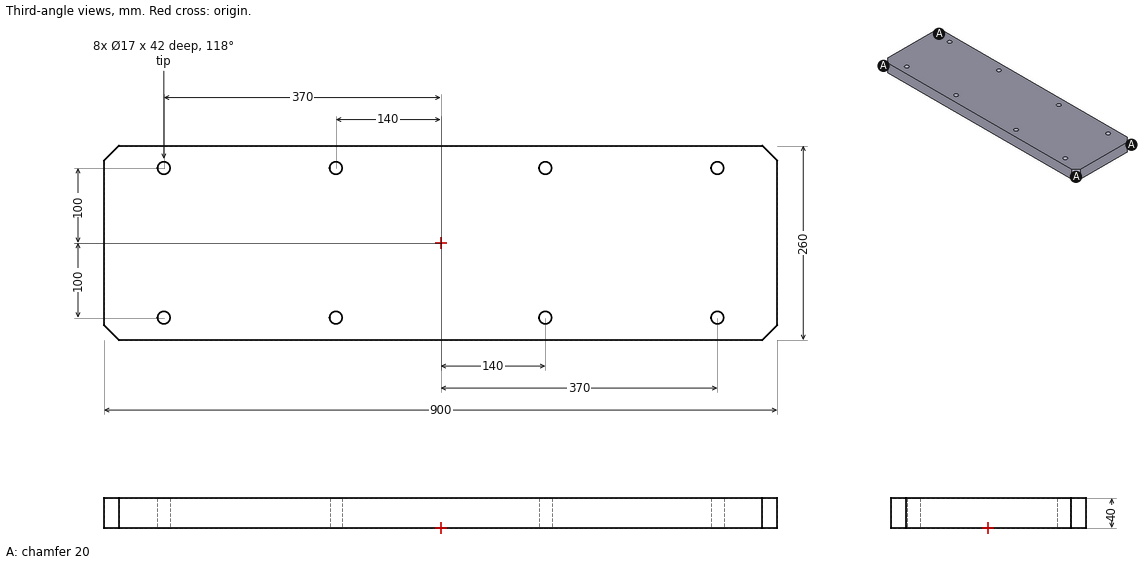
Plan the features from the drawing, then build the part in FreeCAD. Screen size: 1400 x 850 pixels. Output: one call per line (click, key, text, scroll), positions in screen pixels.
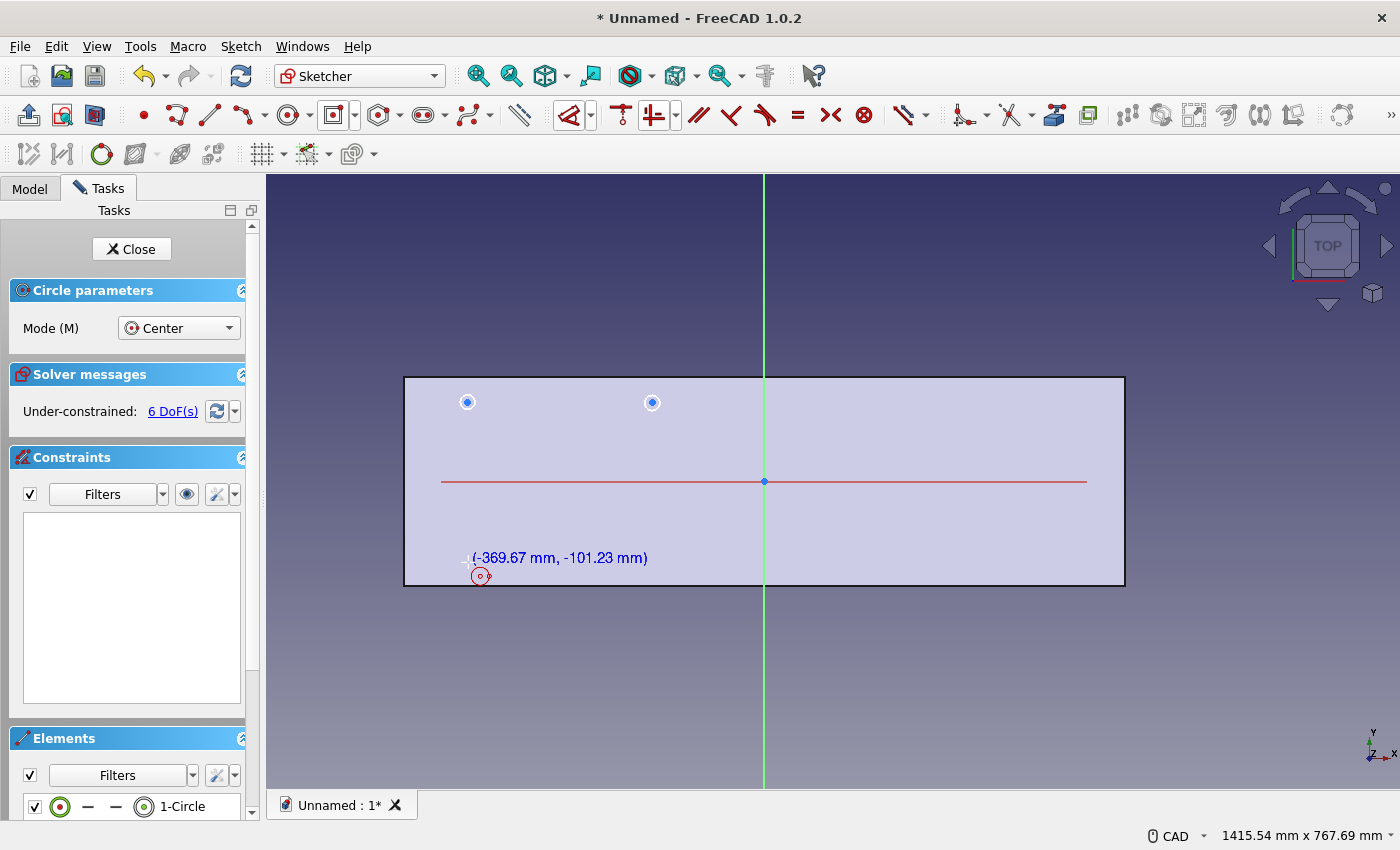
click(468, 562)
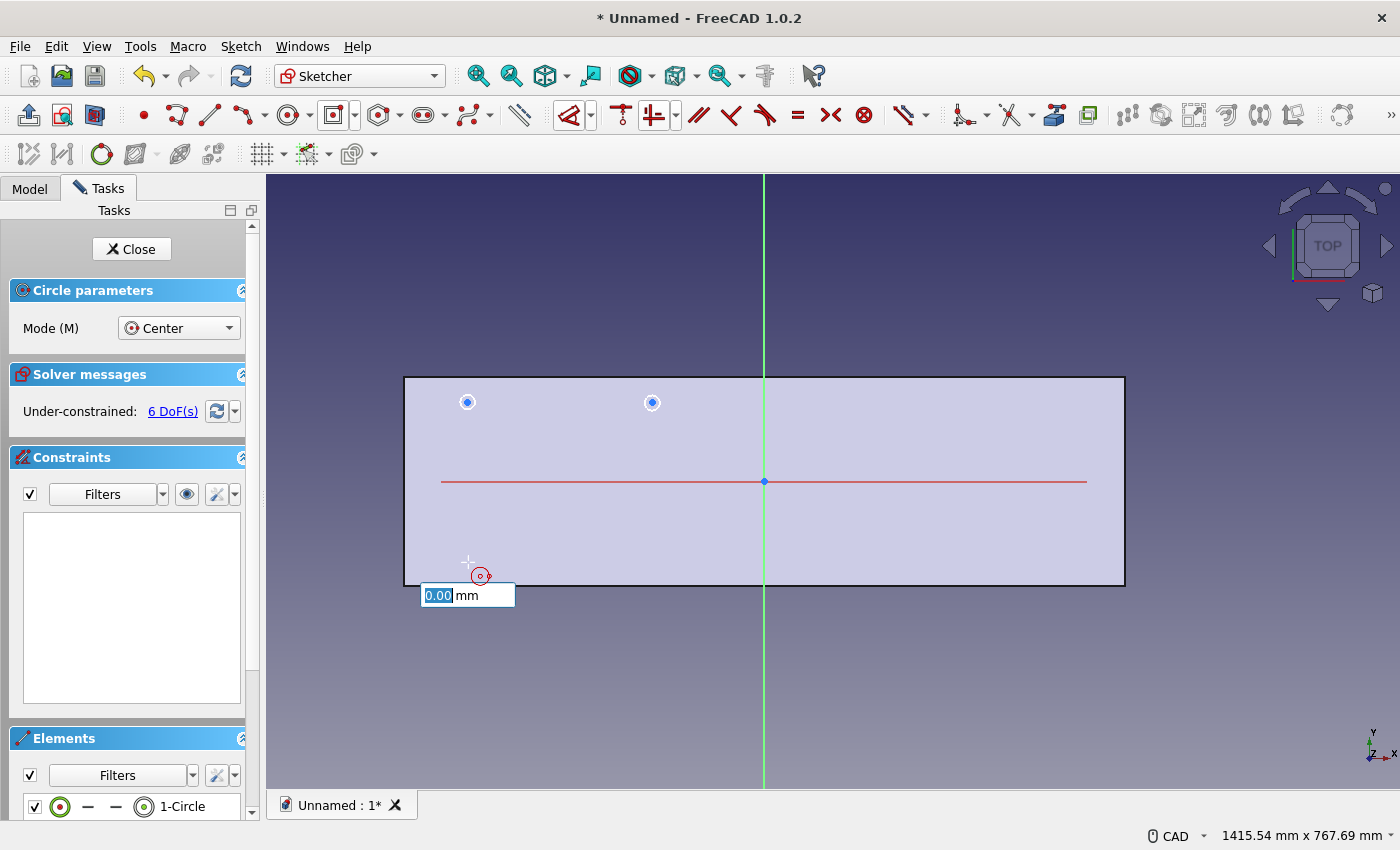
scroll(473, 557, up, 5)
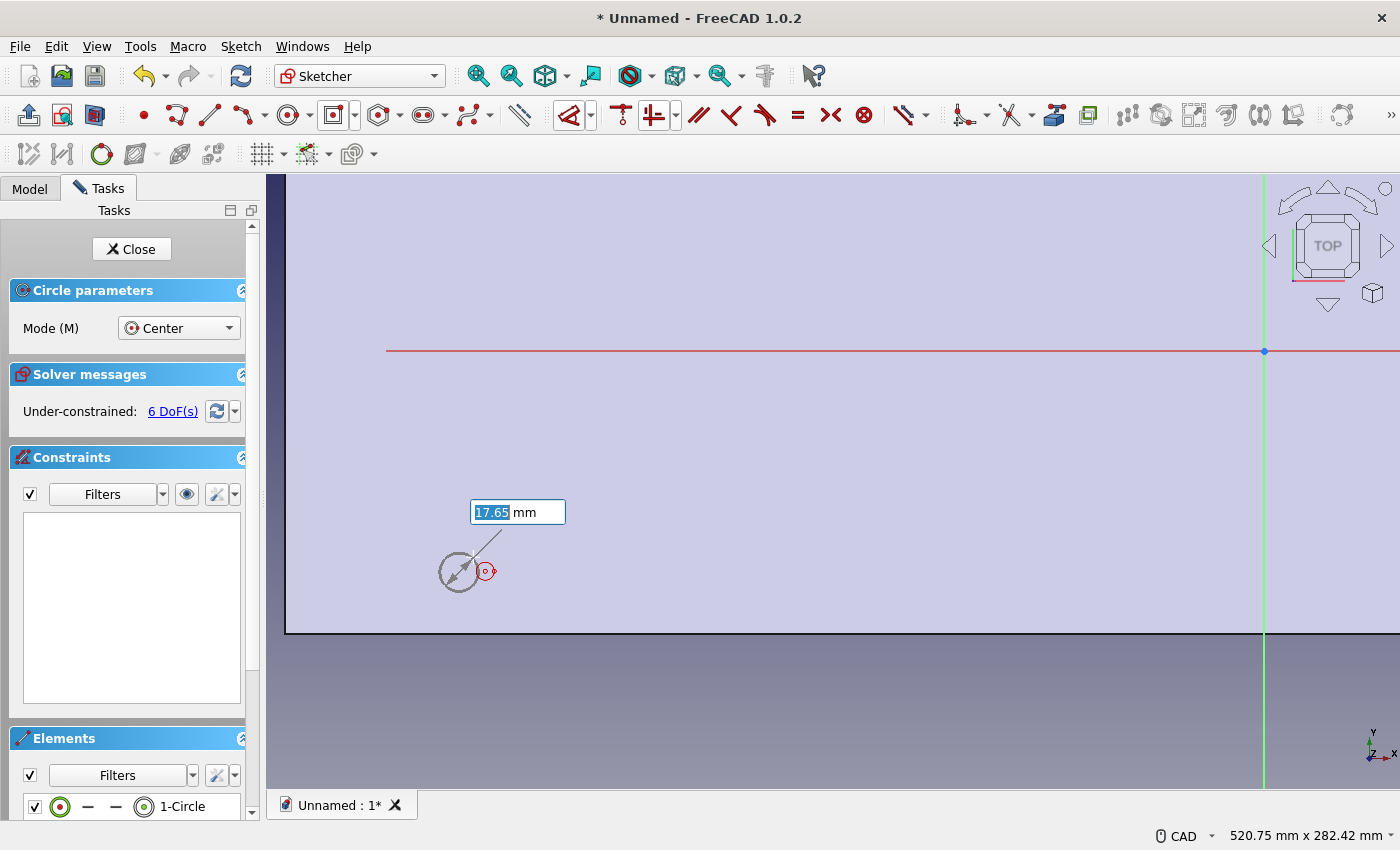
click(472, 556)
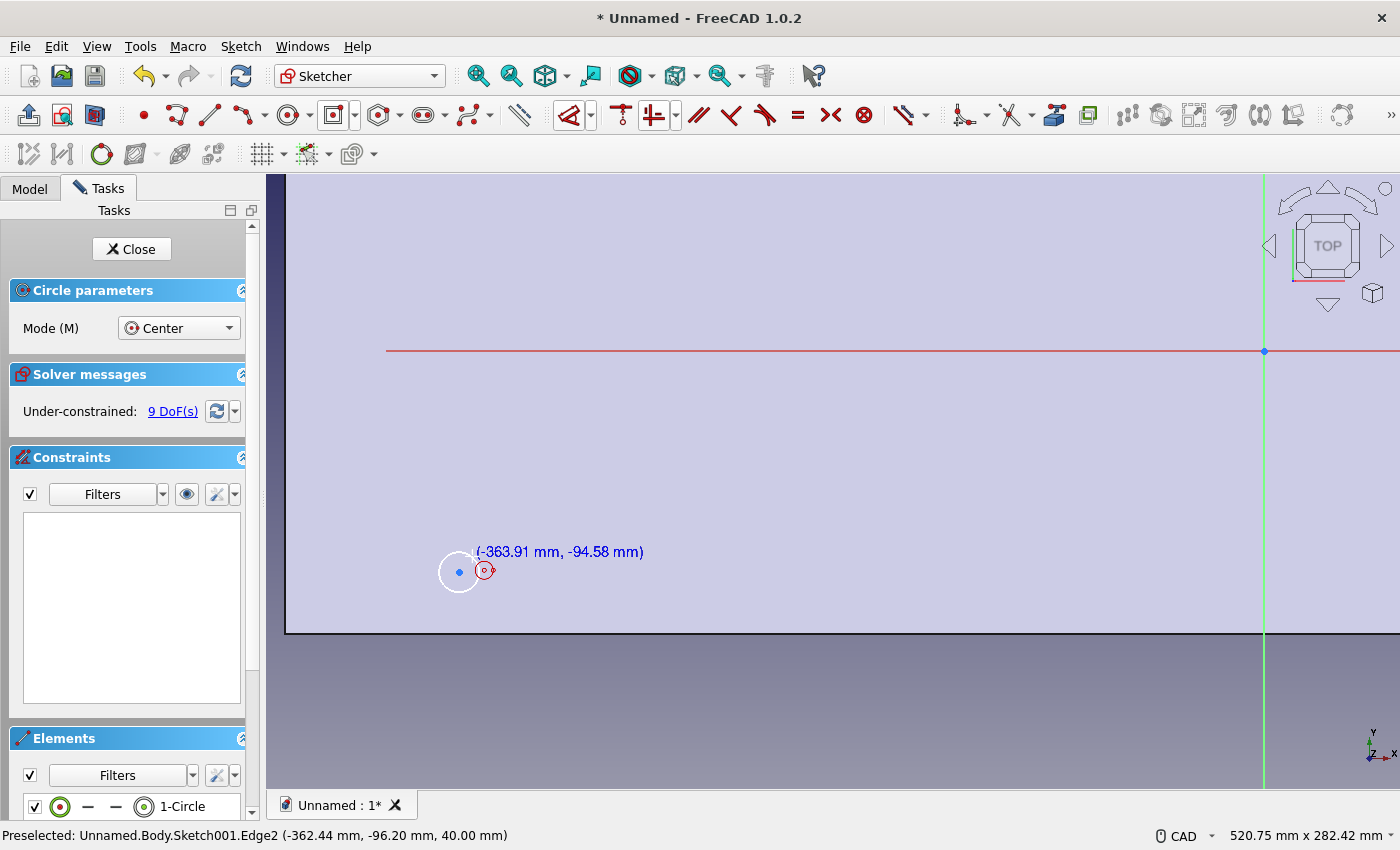
scroll(960, 569, up, 2)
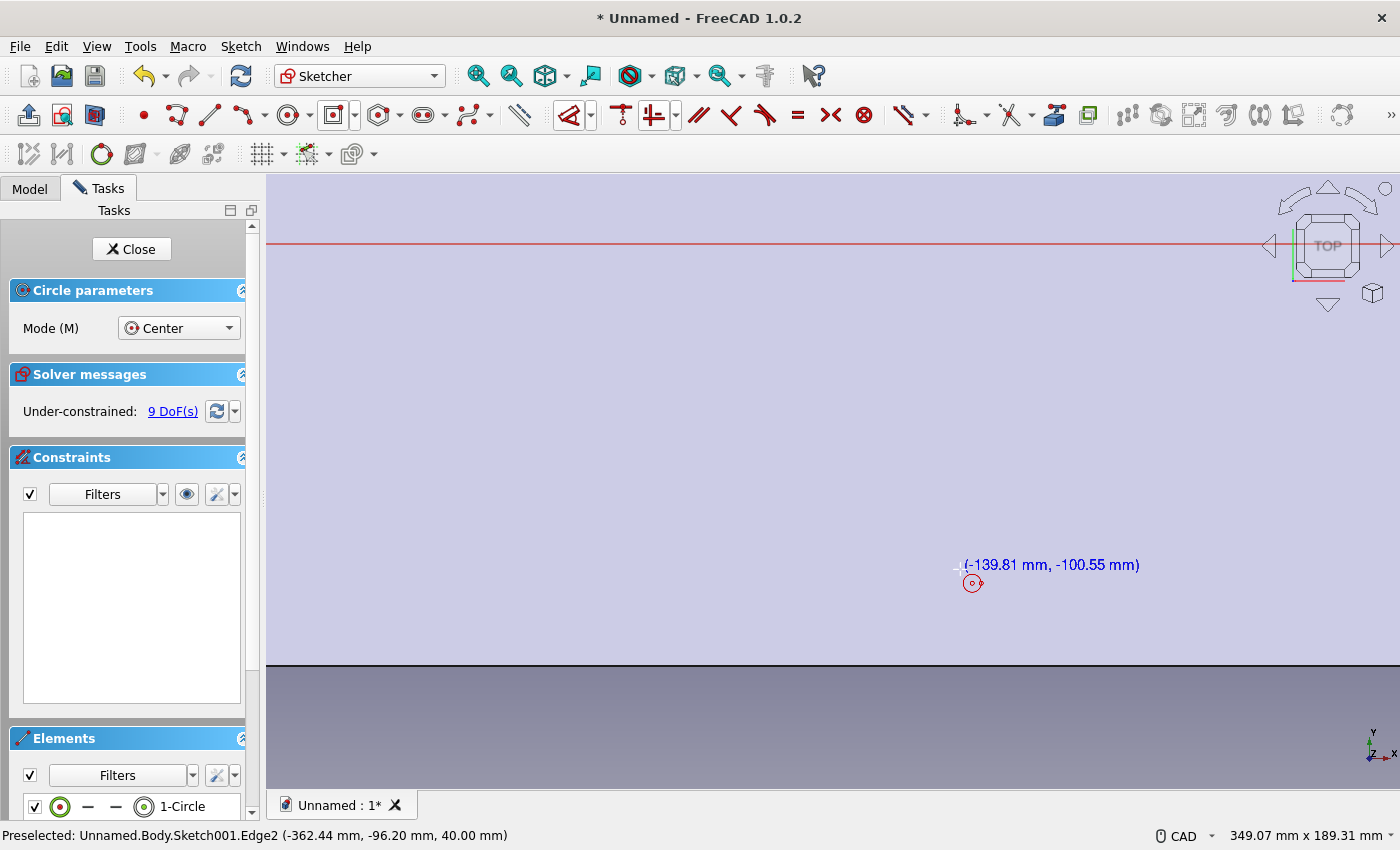
scroll(552, 559, down, 7)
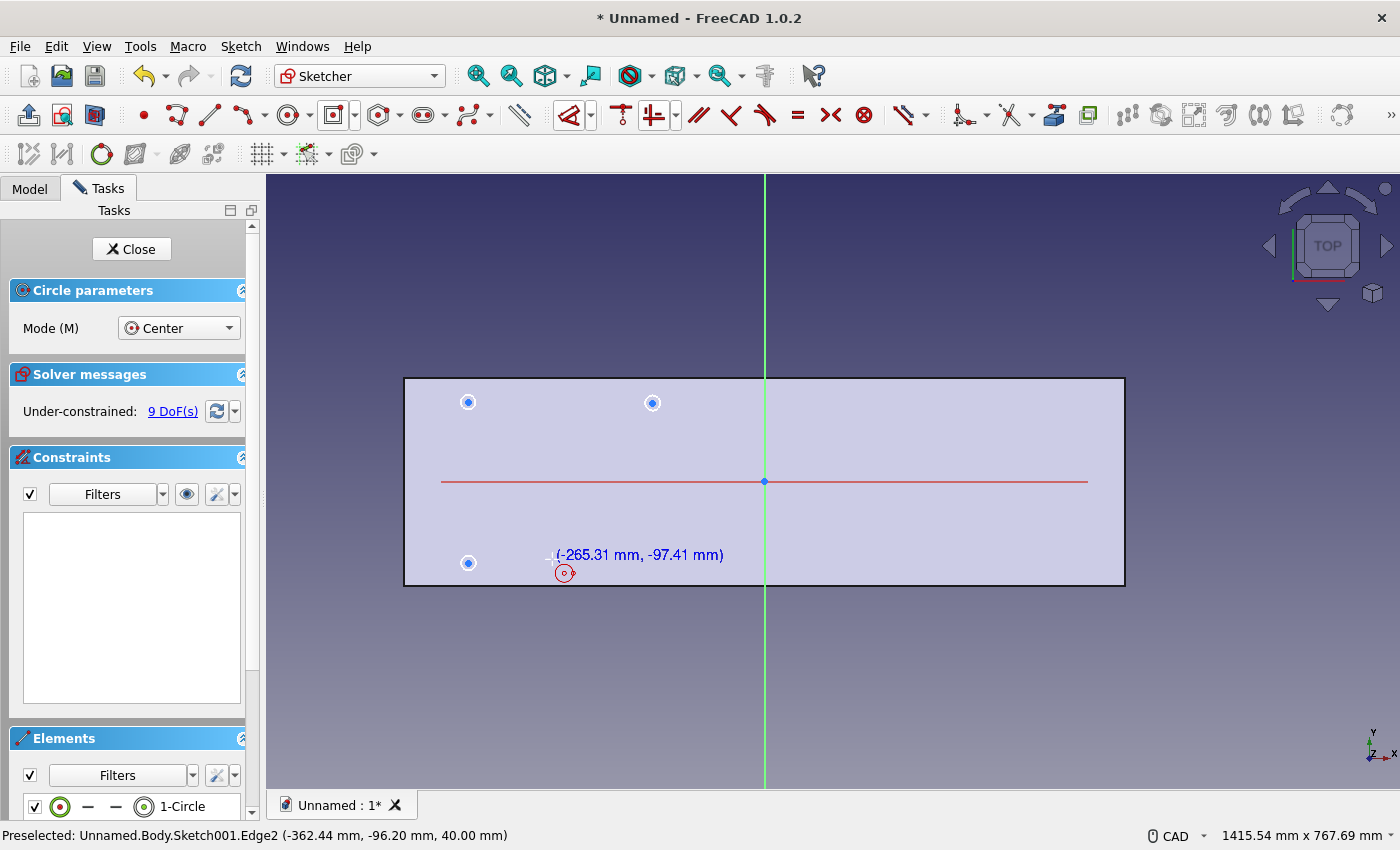
click(653, 562)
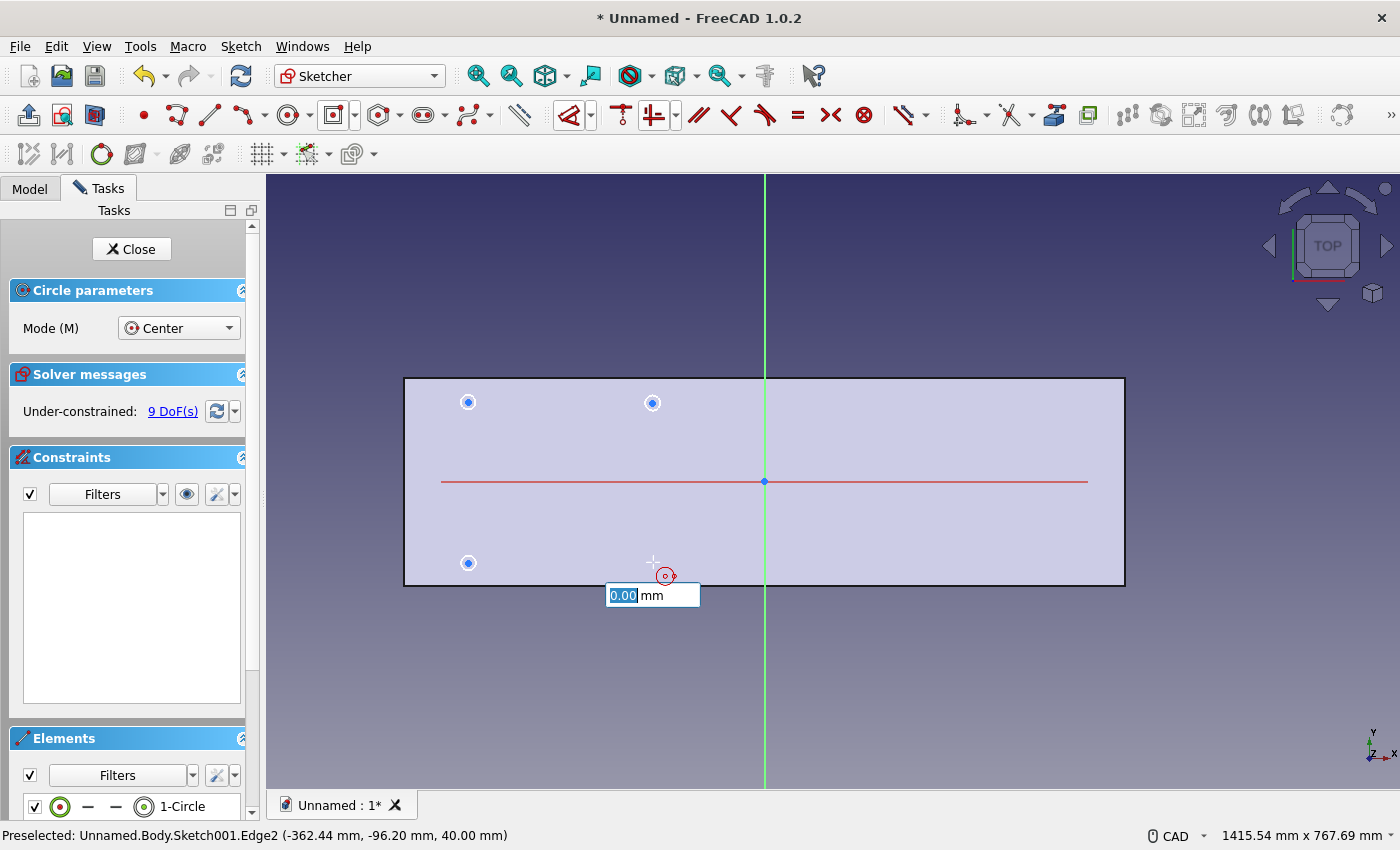
scroll(657, 557, up, 5)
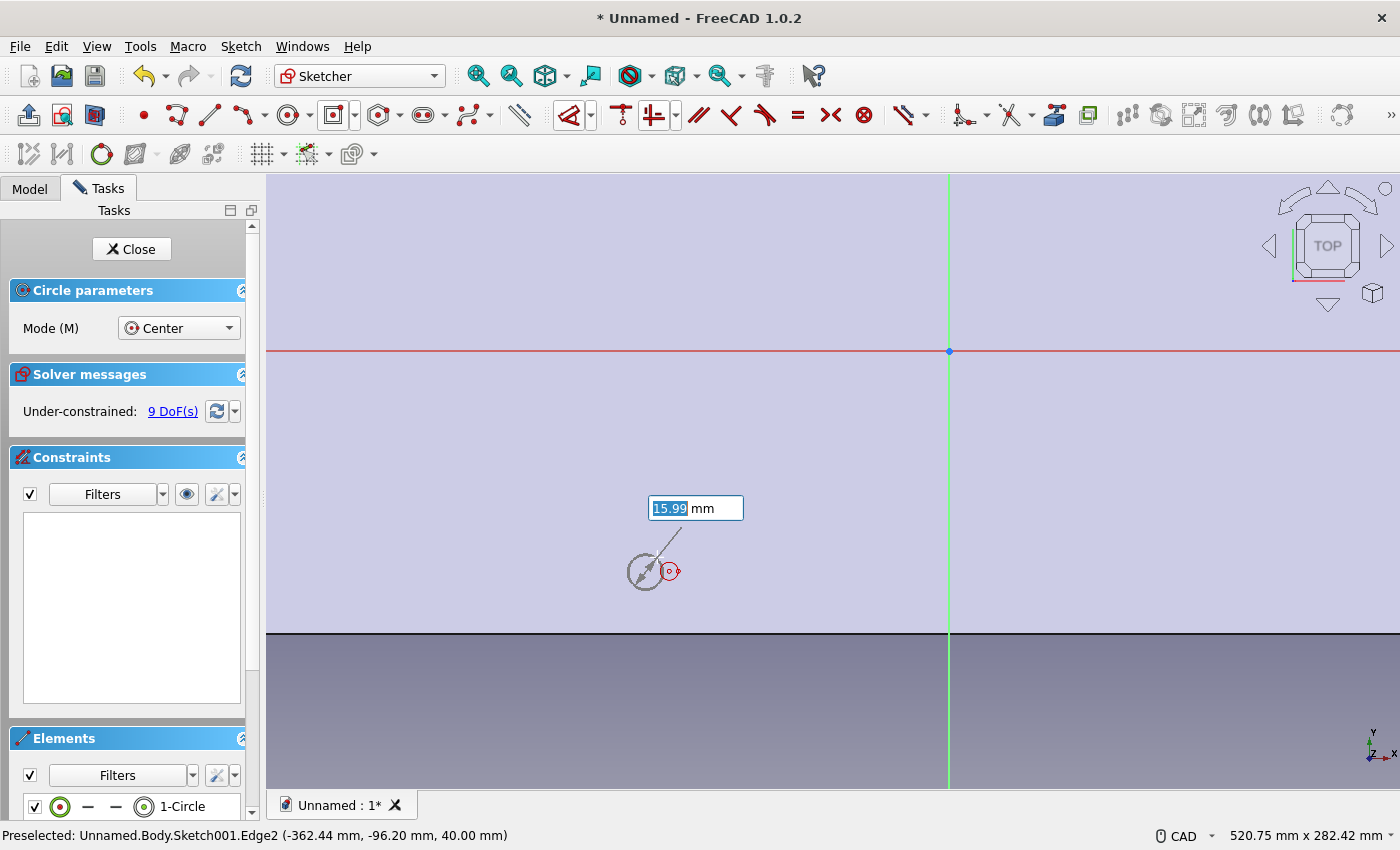
click(657, 556)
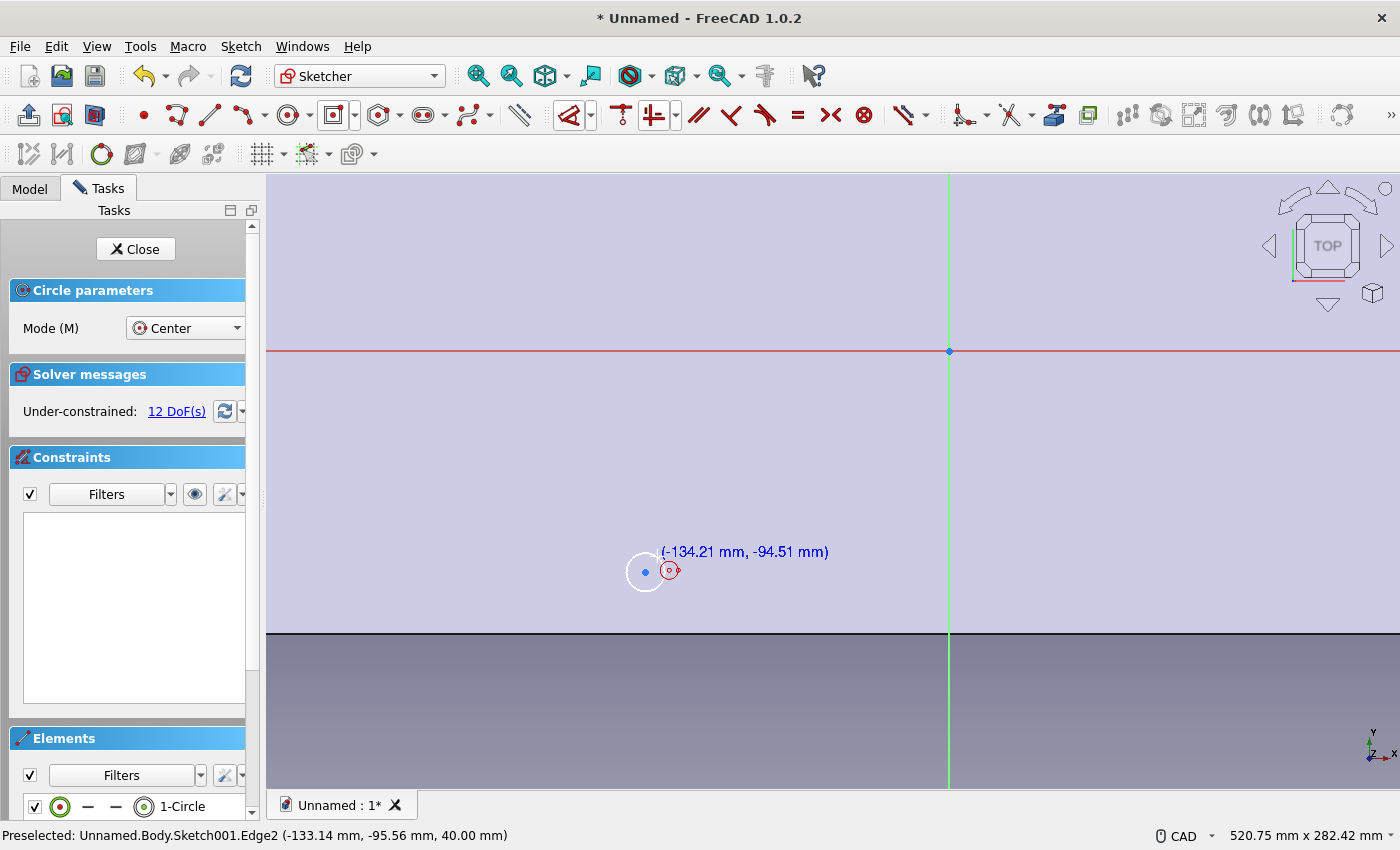
scroll(657, 557, down, 5)